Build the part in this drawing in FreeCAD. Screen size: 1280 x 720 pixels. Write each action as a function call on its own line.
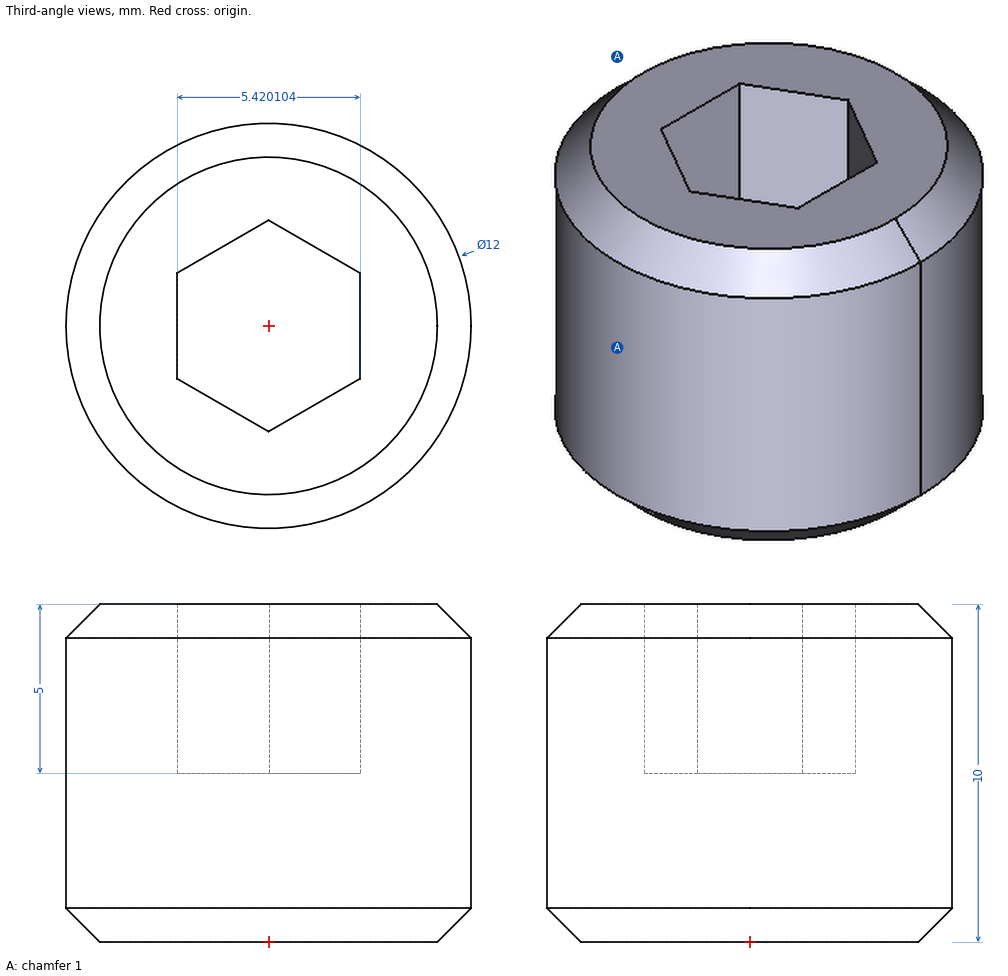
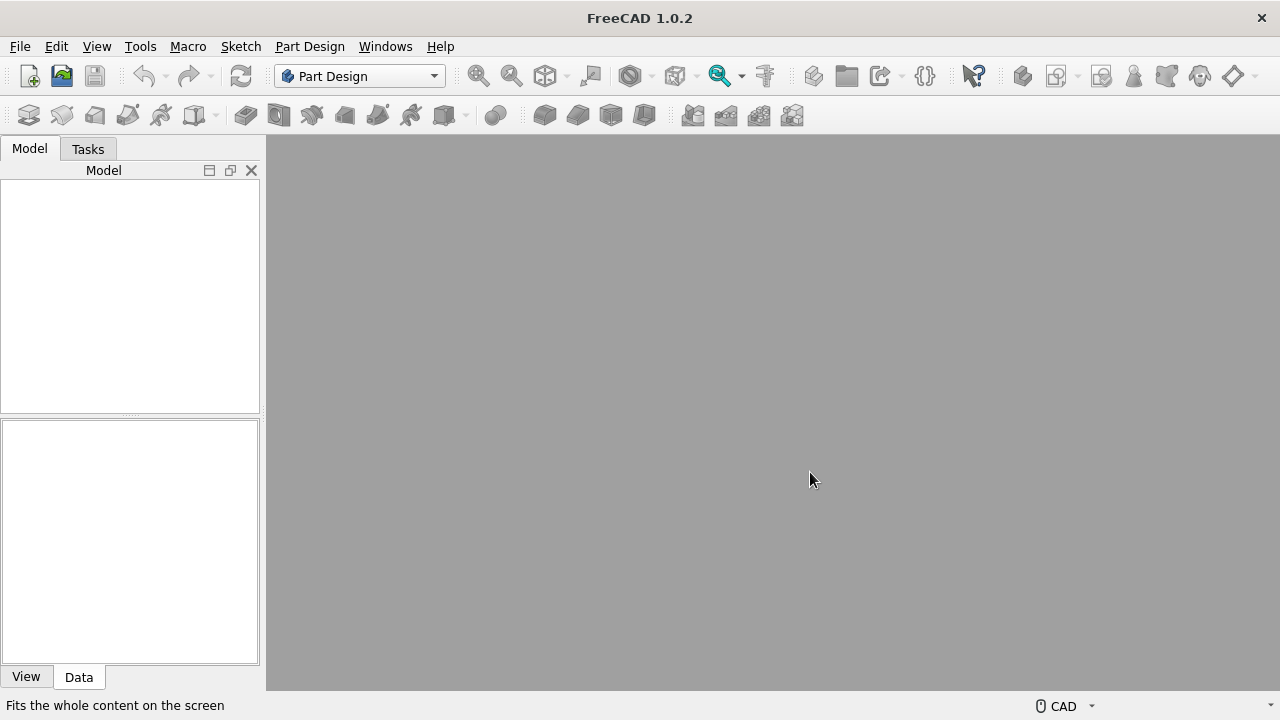
click(29, 76)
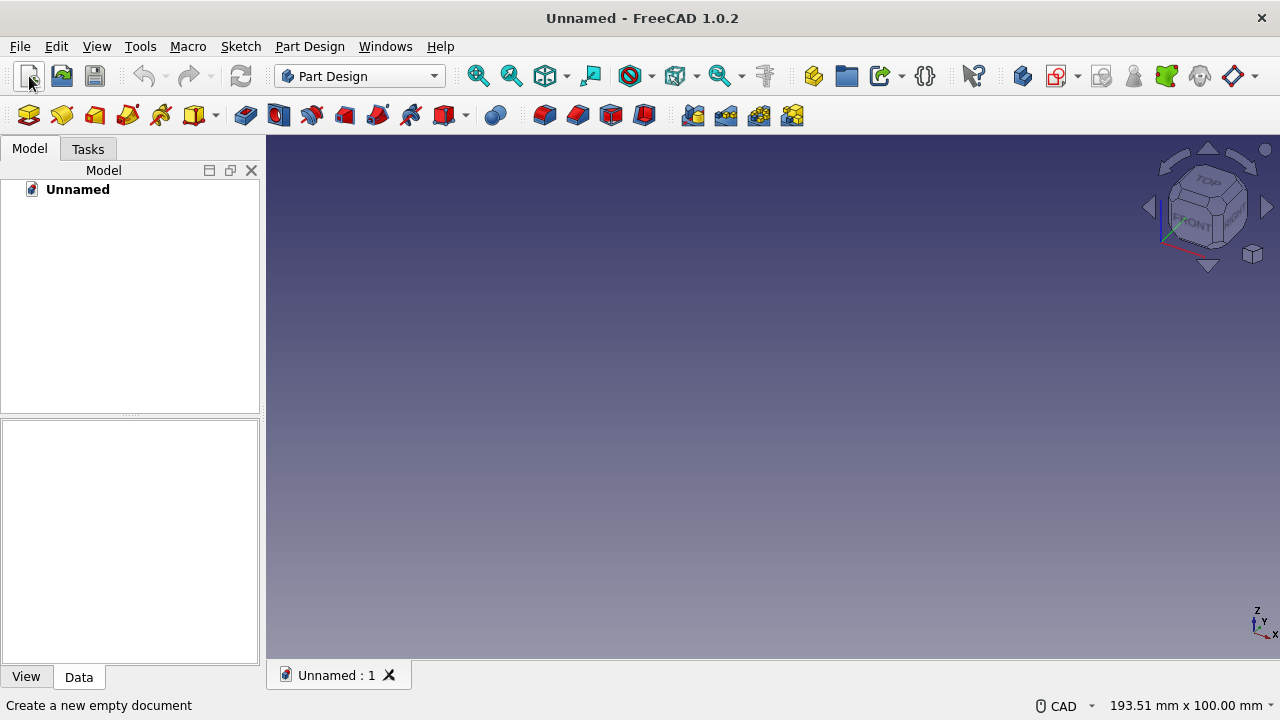
click(1056, 76)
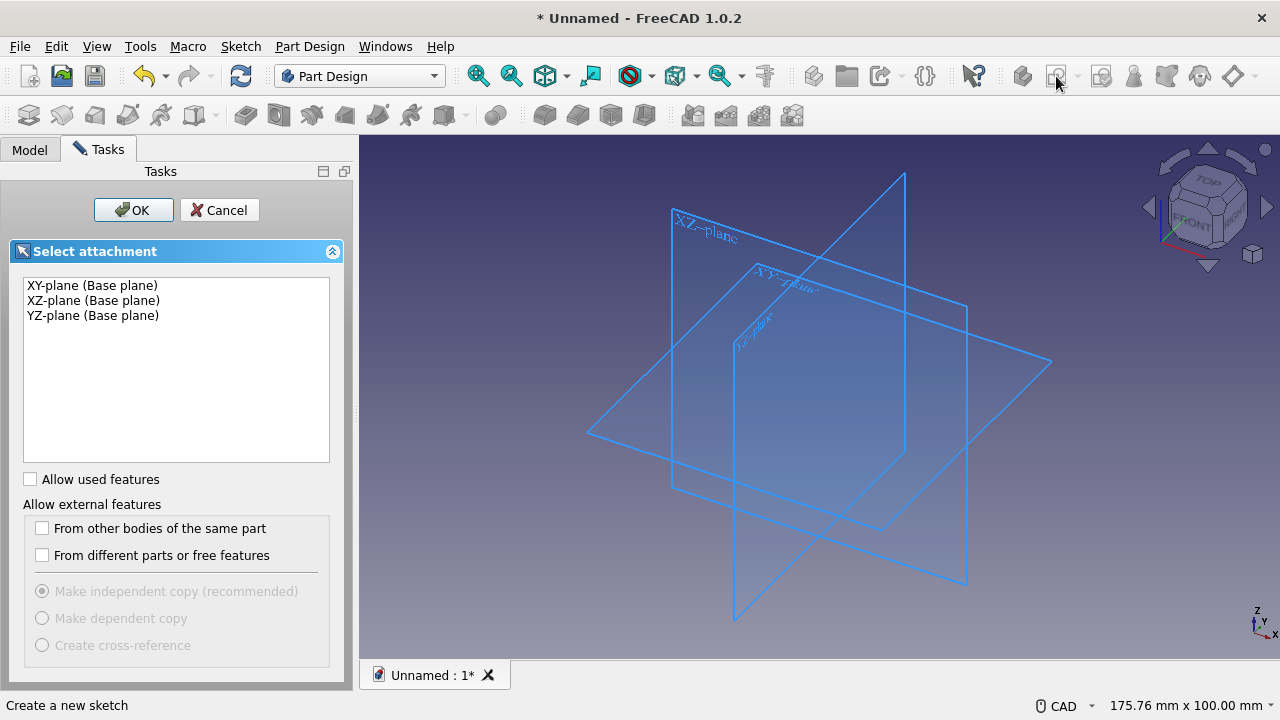
click(84, 286)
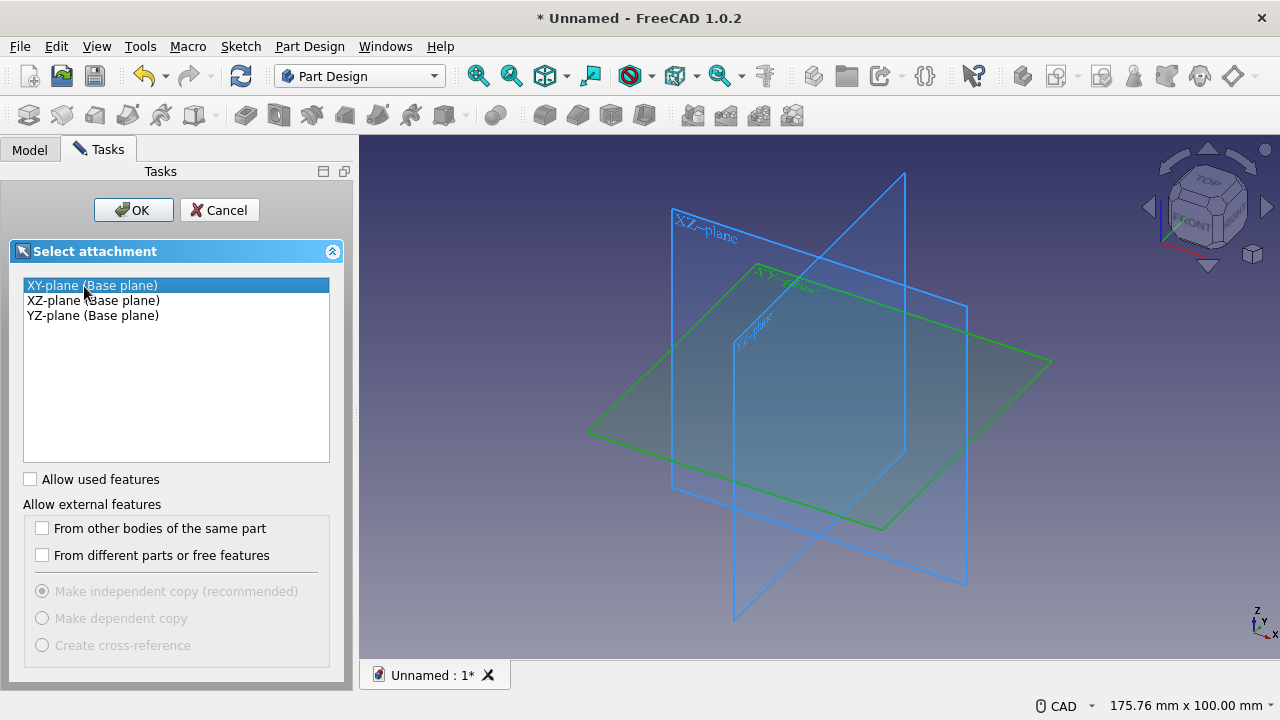
click(134, 210)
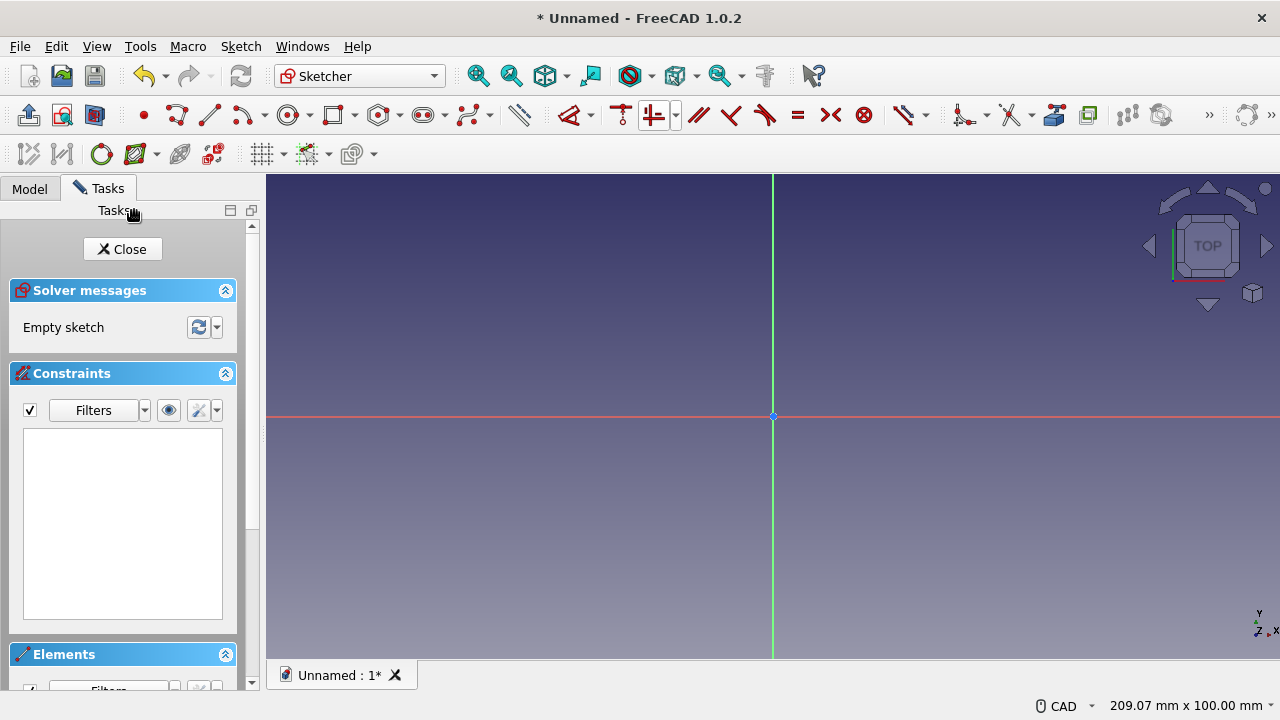
scroll(790, 417, up, 8)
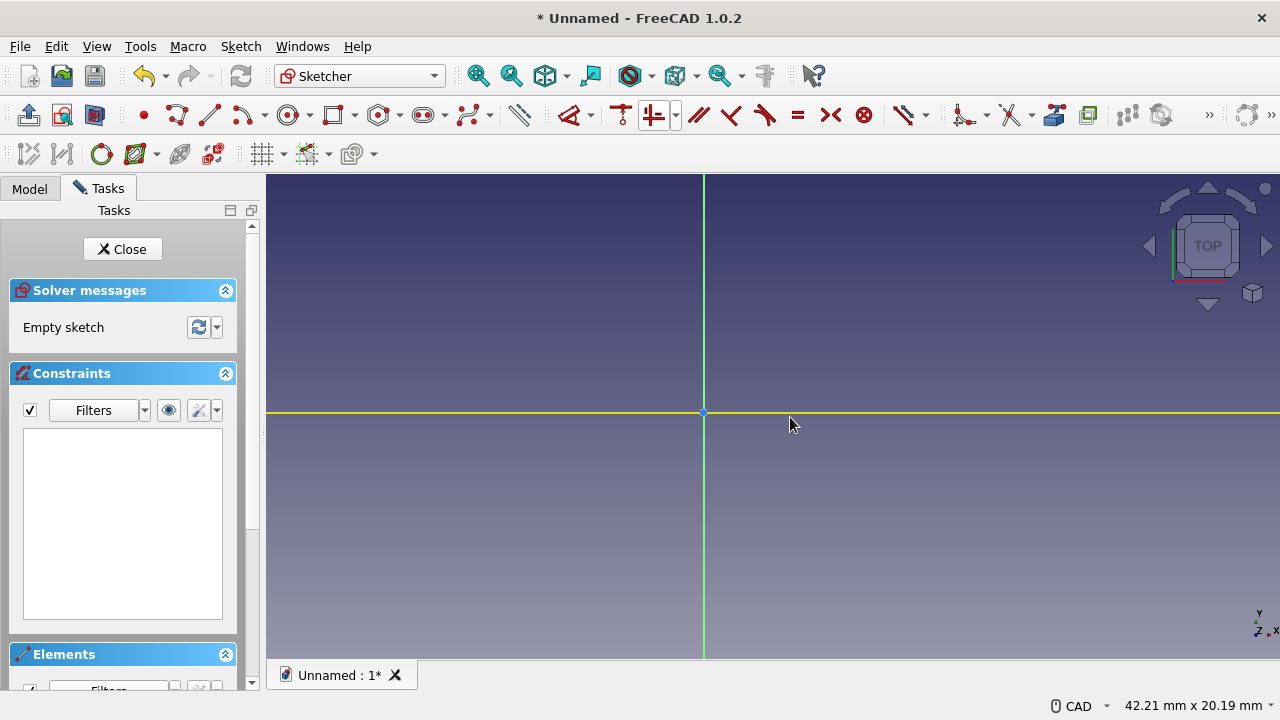
click(288, 116)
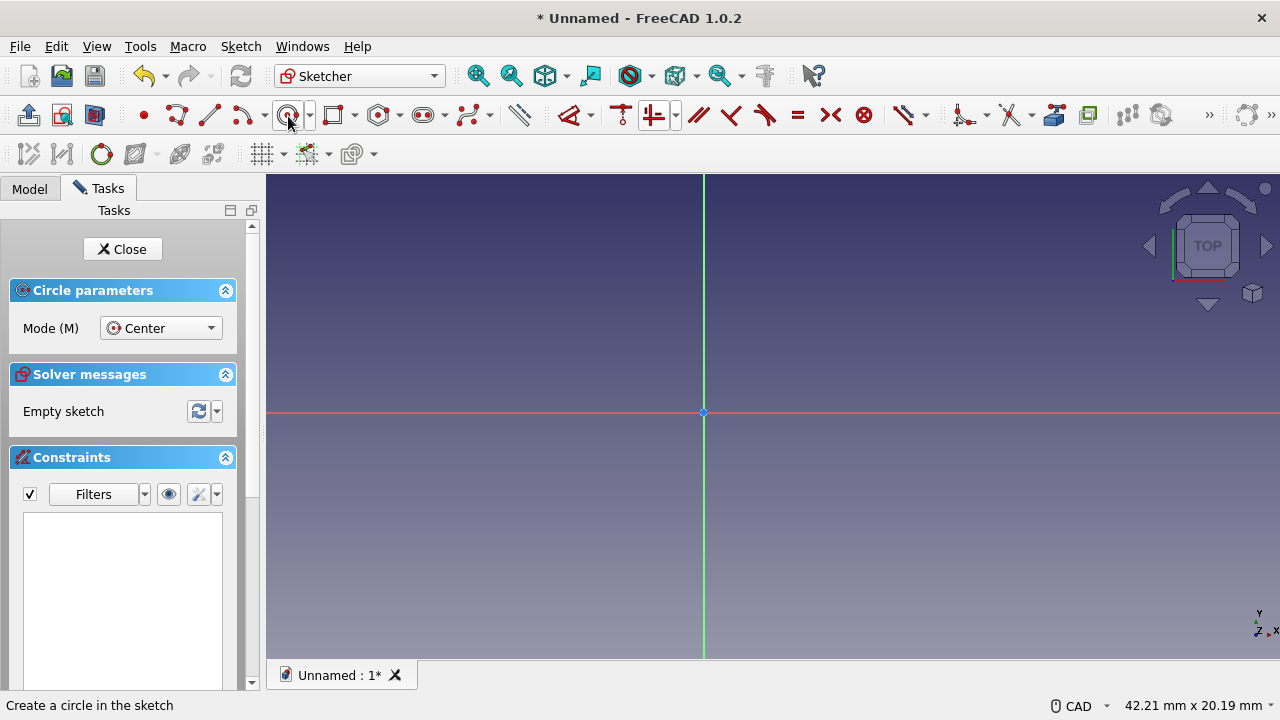
click(704, 413)
click(806, 311)
key(Escape)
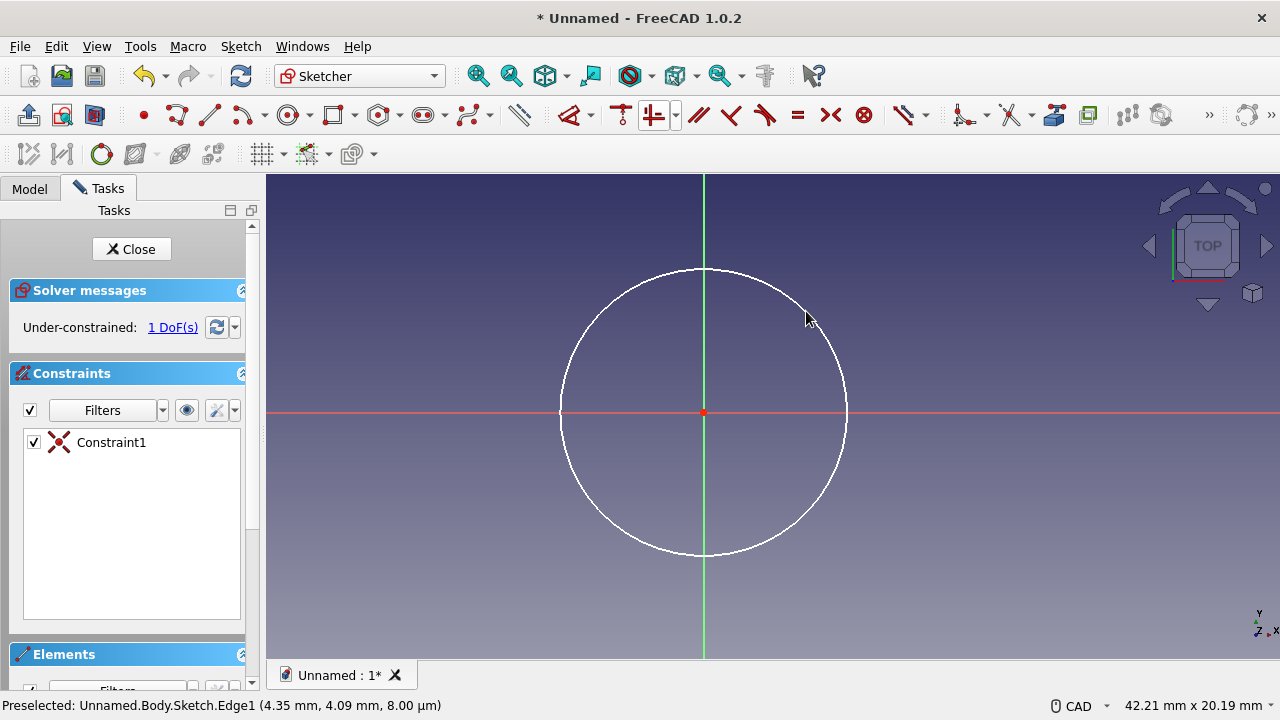
click(805, 311)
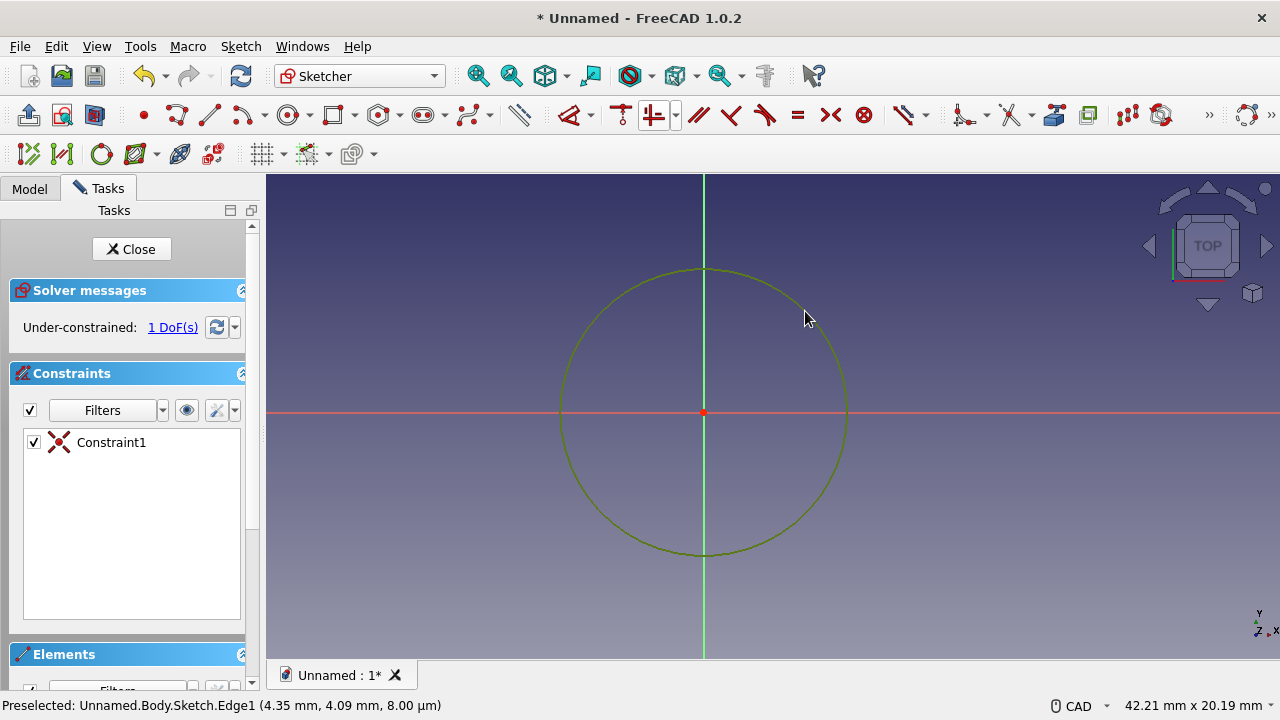
key(k)
key(o)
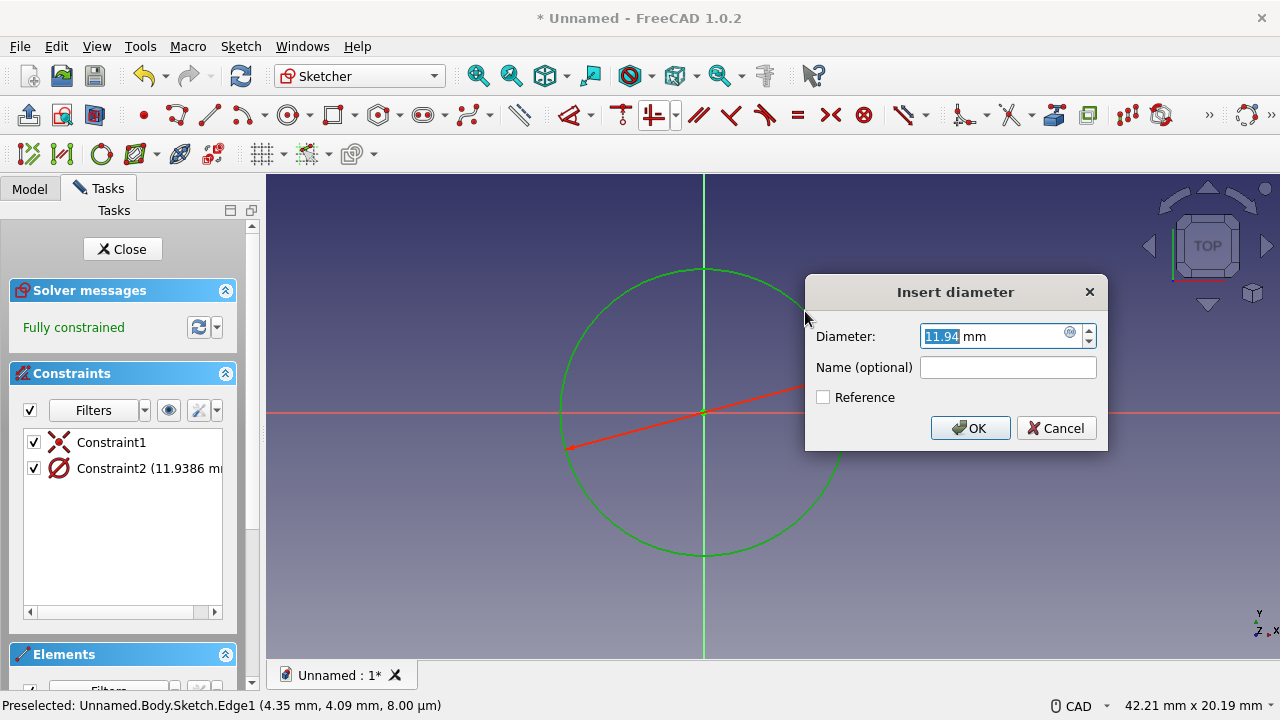
text(12)
key(Return)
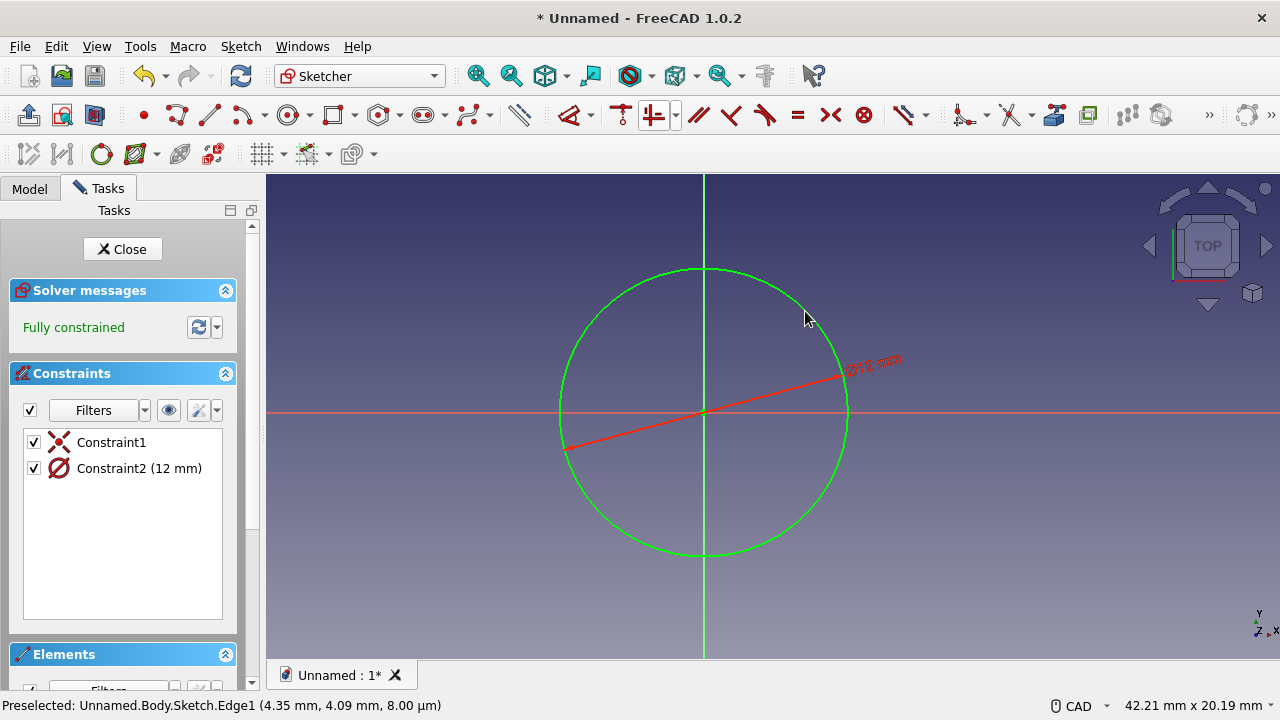
click(123, 249)